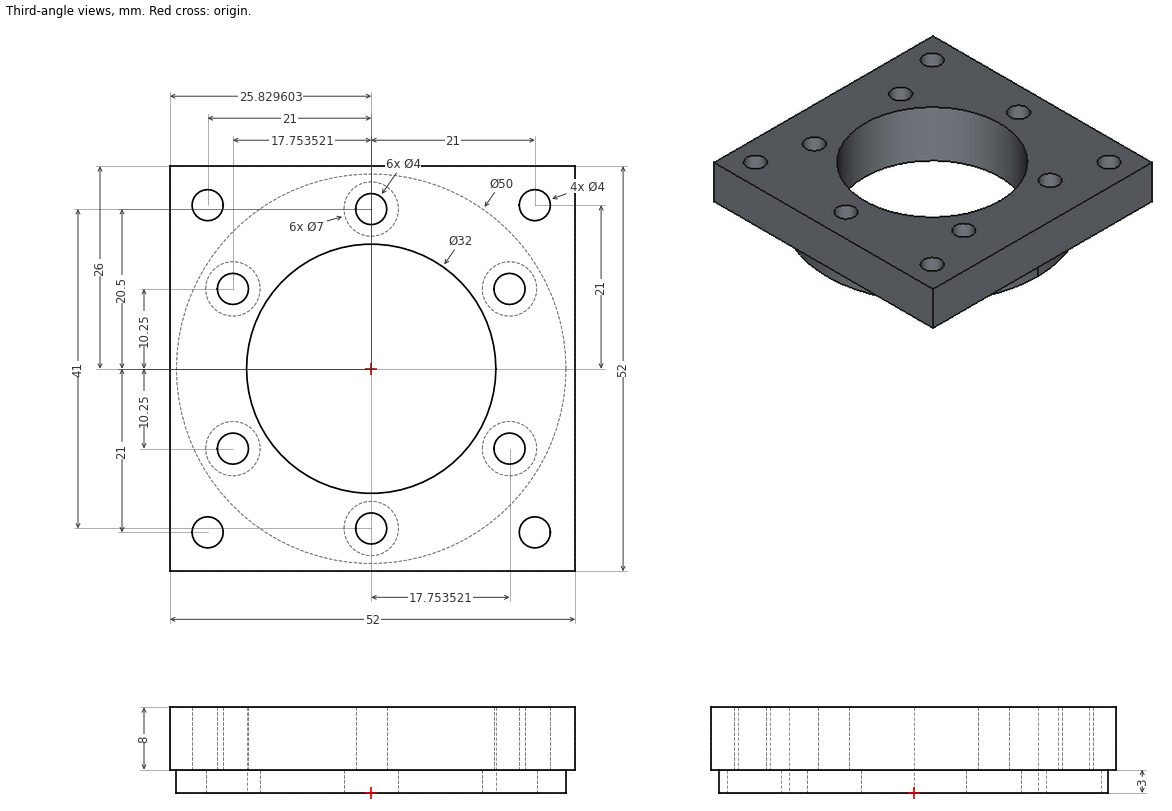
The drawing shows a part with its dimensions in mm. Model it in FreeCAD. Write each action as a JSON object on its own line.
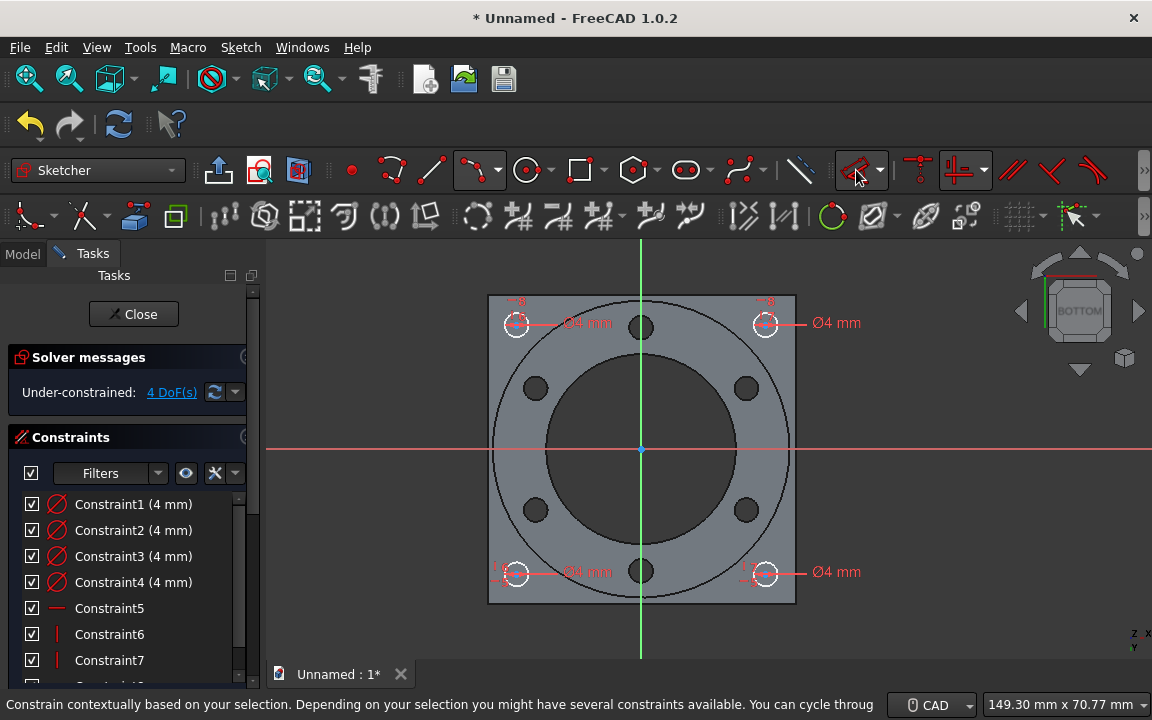
{"action": "left_click", "coordinate": [766, 574]}
{"action": "left_click", "coordinate": [703, 608]}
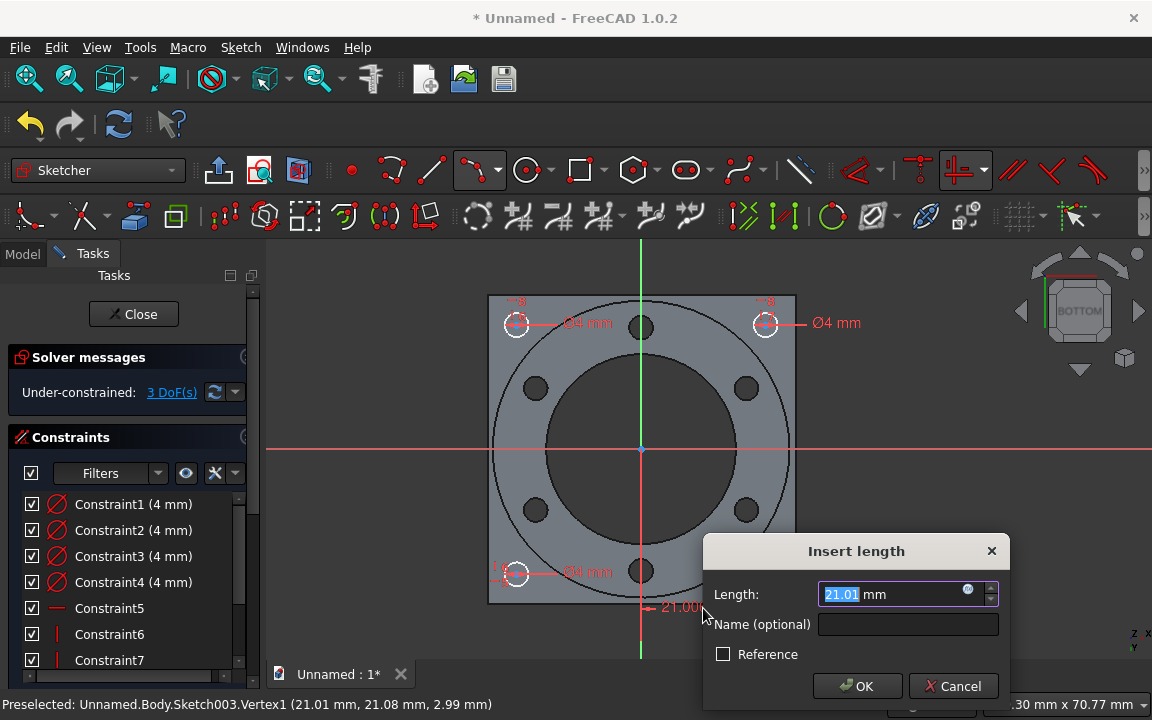
{"action": "type", "text": "21"}
{"action": "key", "text": "Return"}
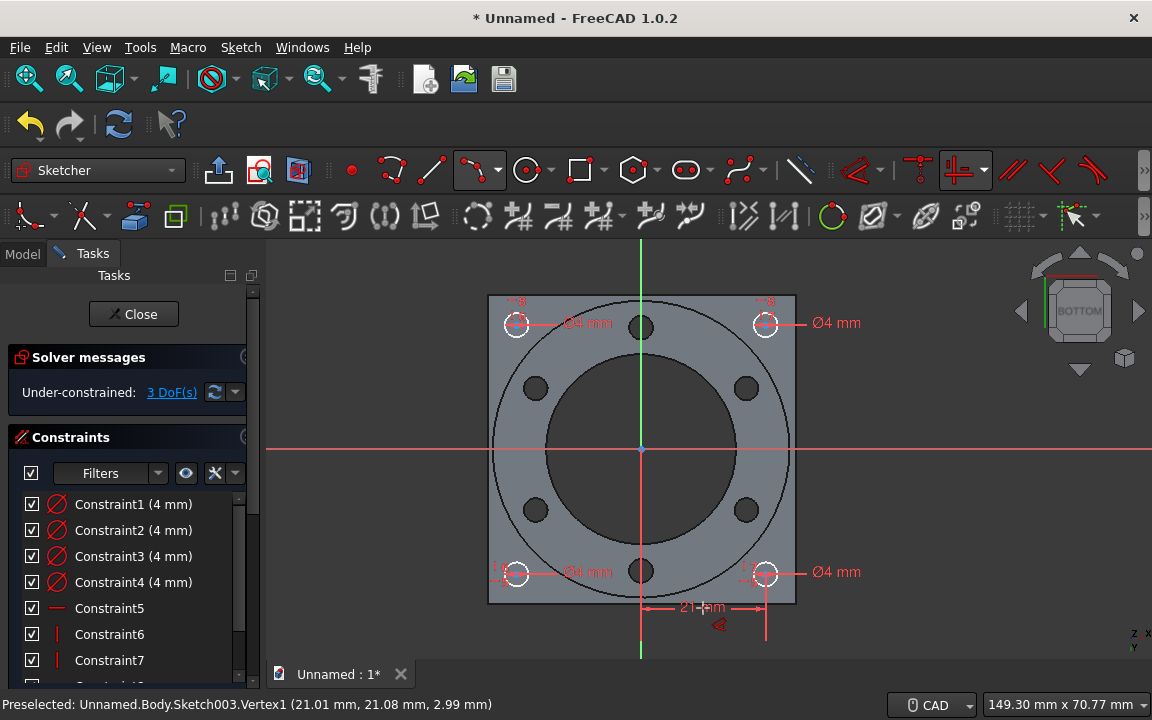
{"action": "left_click", "coordinate": [766, 574]}
{"action": "left_click", "coordinate": [800, 512]}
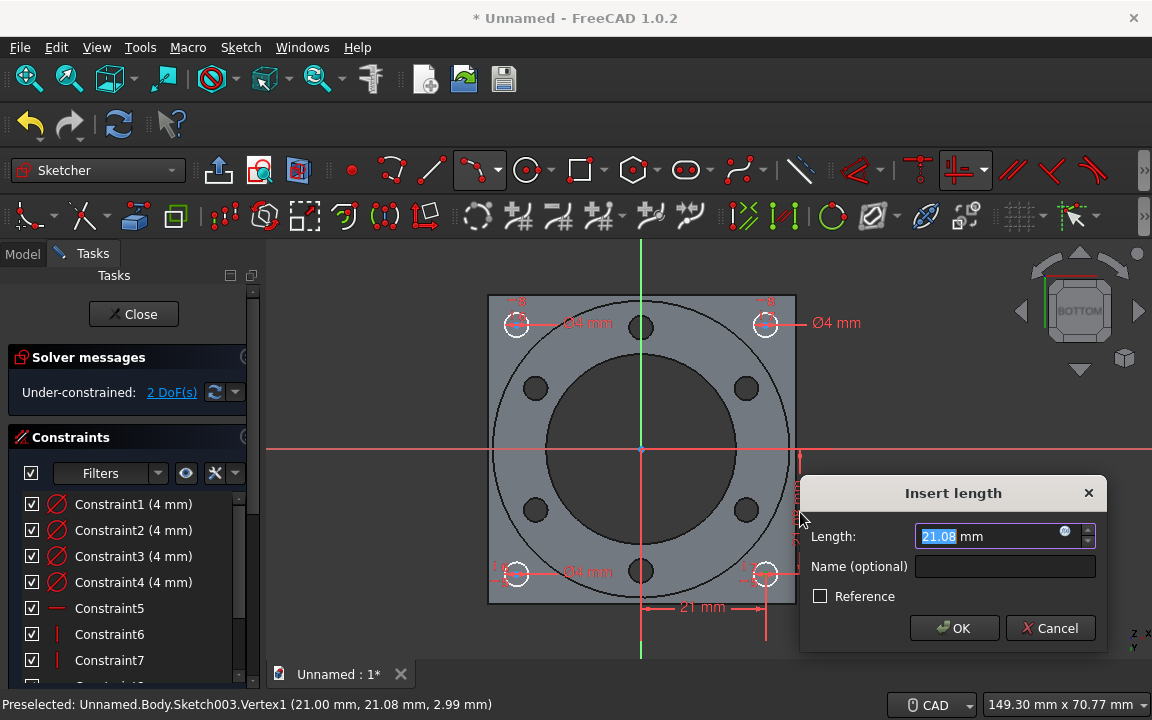
{"action": "type", "text": "21"}
{"action": "key", "text": "Return"}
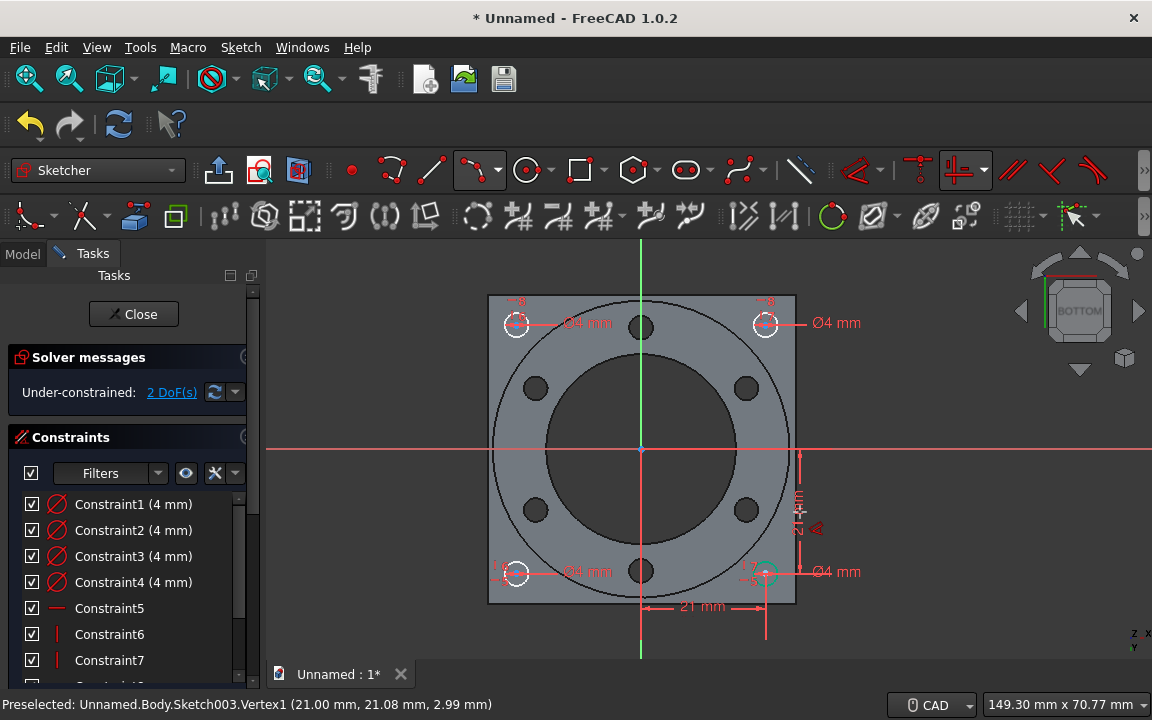
{"action": "left_click", "coordinate": [517, 574]}
{"action": "left_click", "coordinate": [579, 608]}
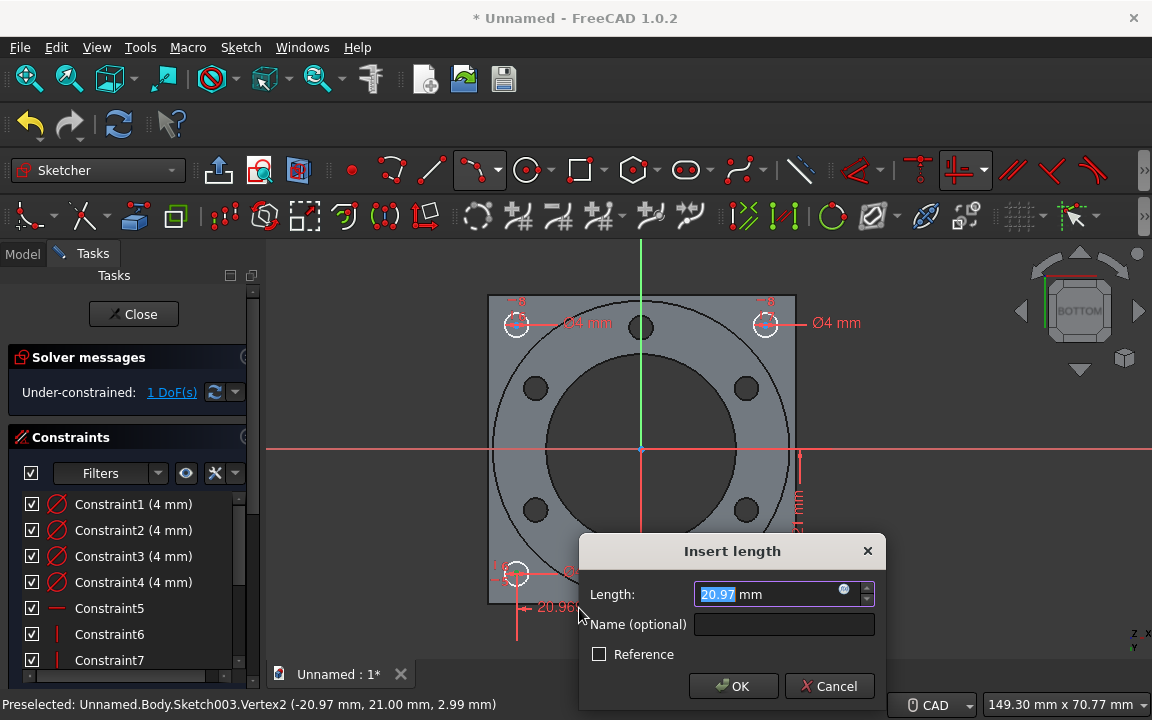
{"action": "type", "text": "21"}
{"action": "key", "text": "Return"}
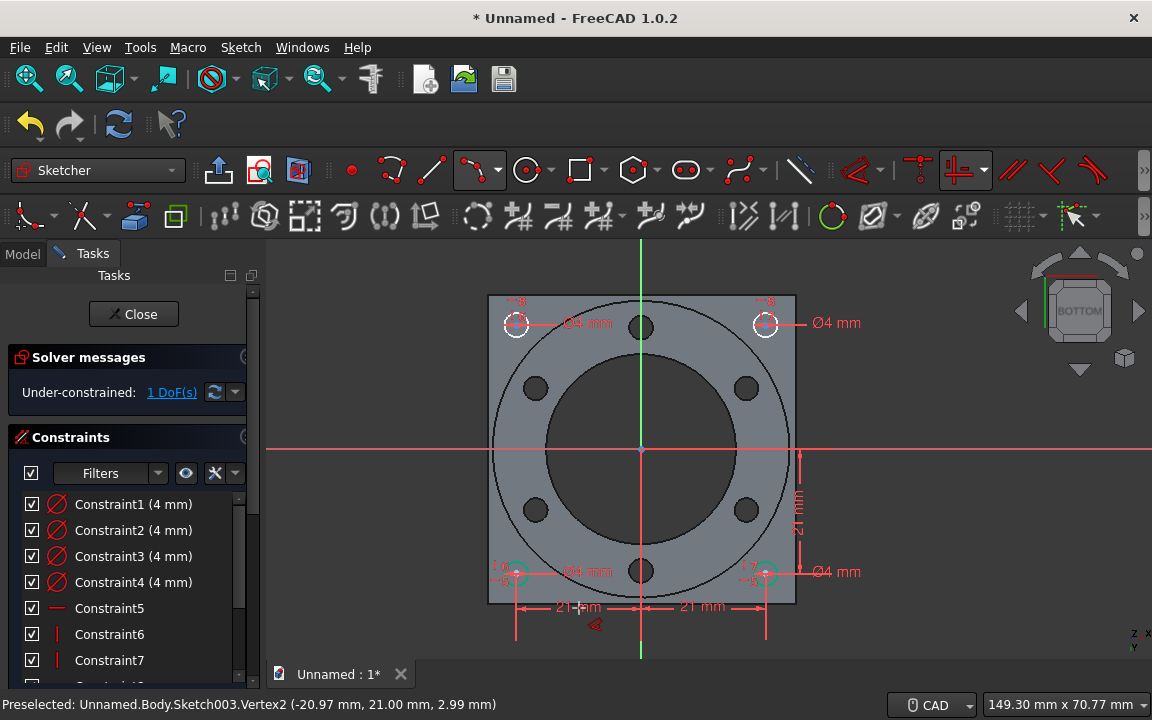
{"action": "left_click", "coordinate": [516, 325]}
{"action": "left_click", "coordinate": [482, 387]}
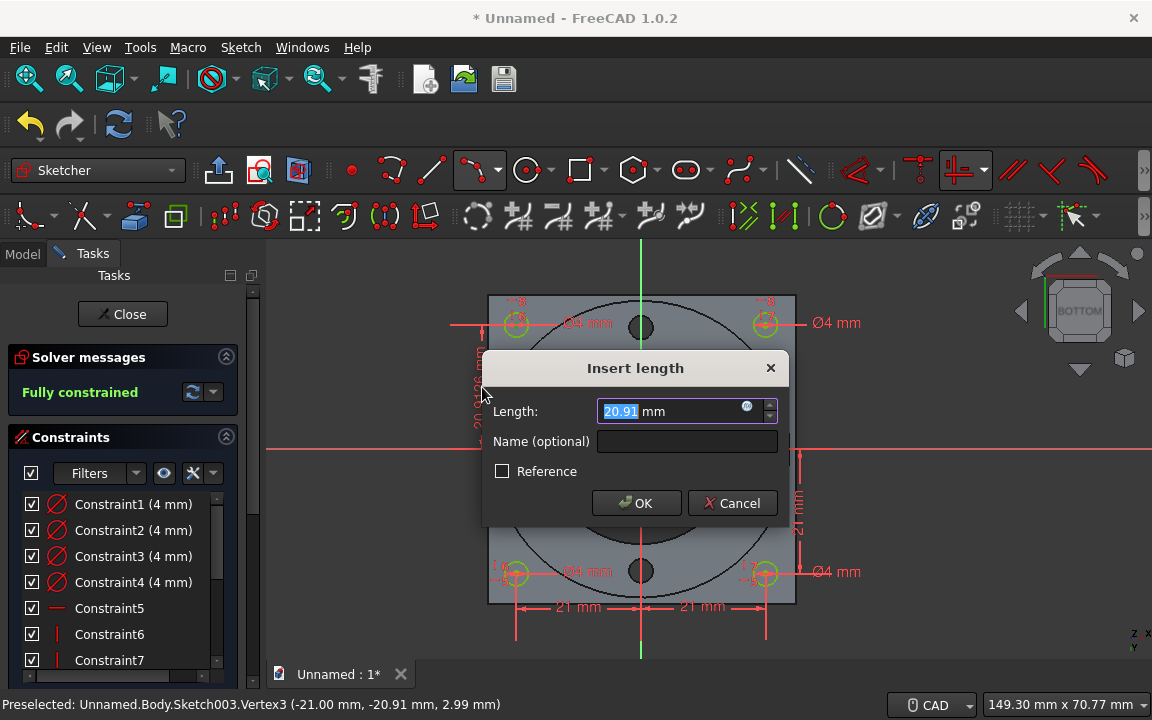
{"action": "type", "text": "21"}
{"action": "key", "text": "Return"}
{"action": "key", "text": "Escape"}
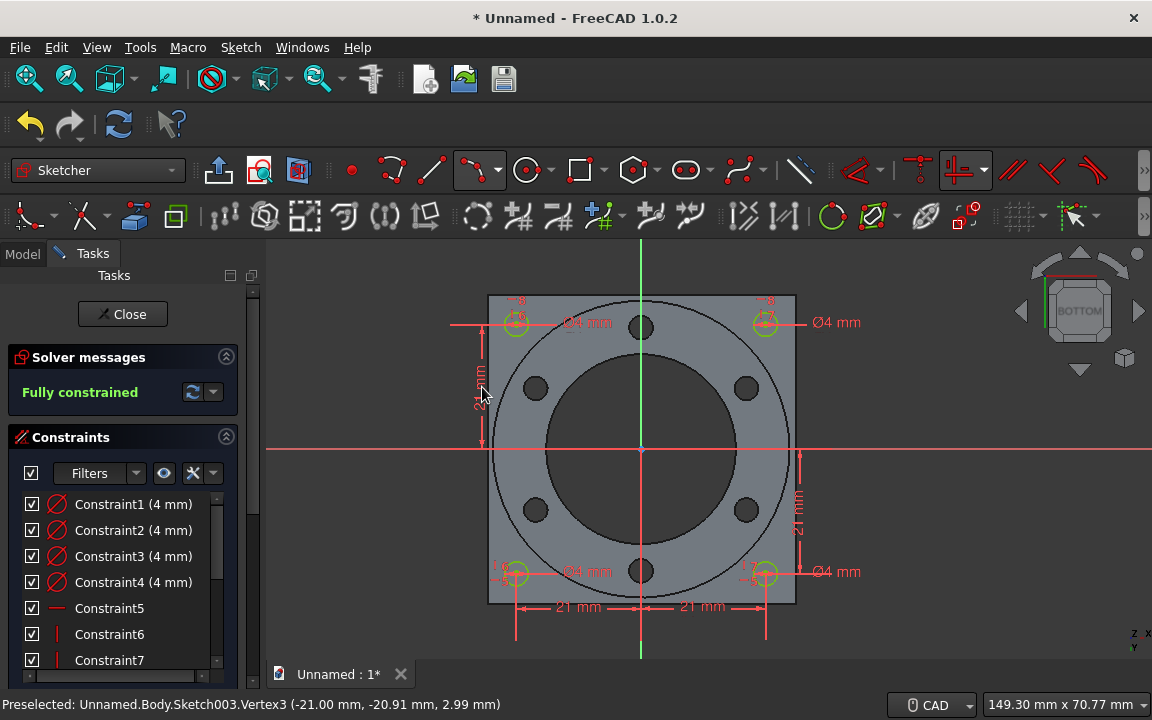
{"action": "left_click", "coordinate": [123, 314]}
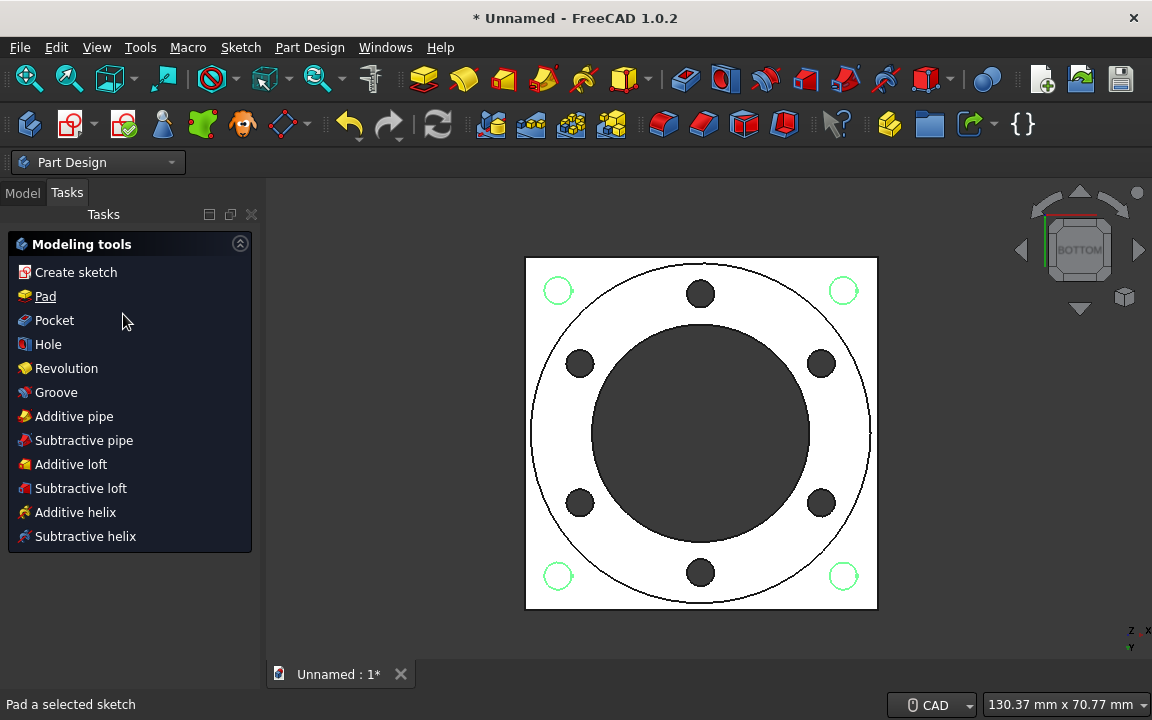
{"action": "left_click", "coordinate": [686, 80]}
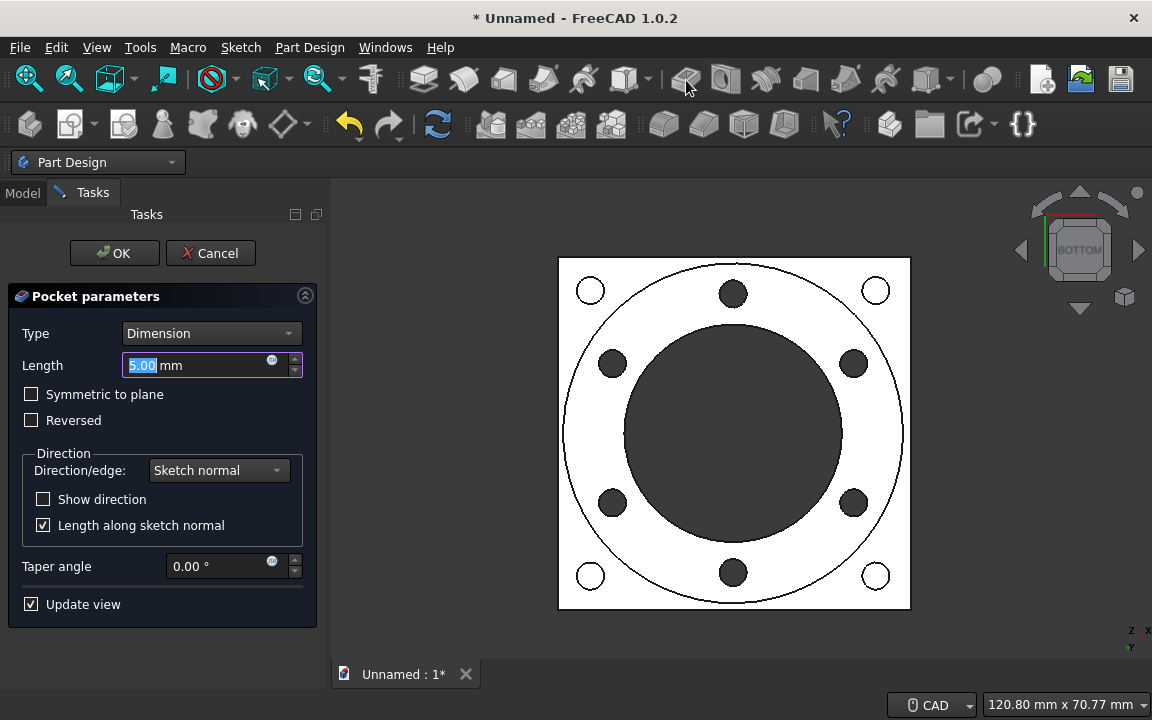
{"action": "left_click", "coordinate": [212, 334]}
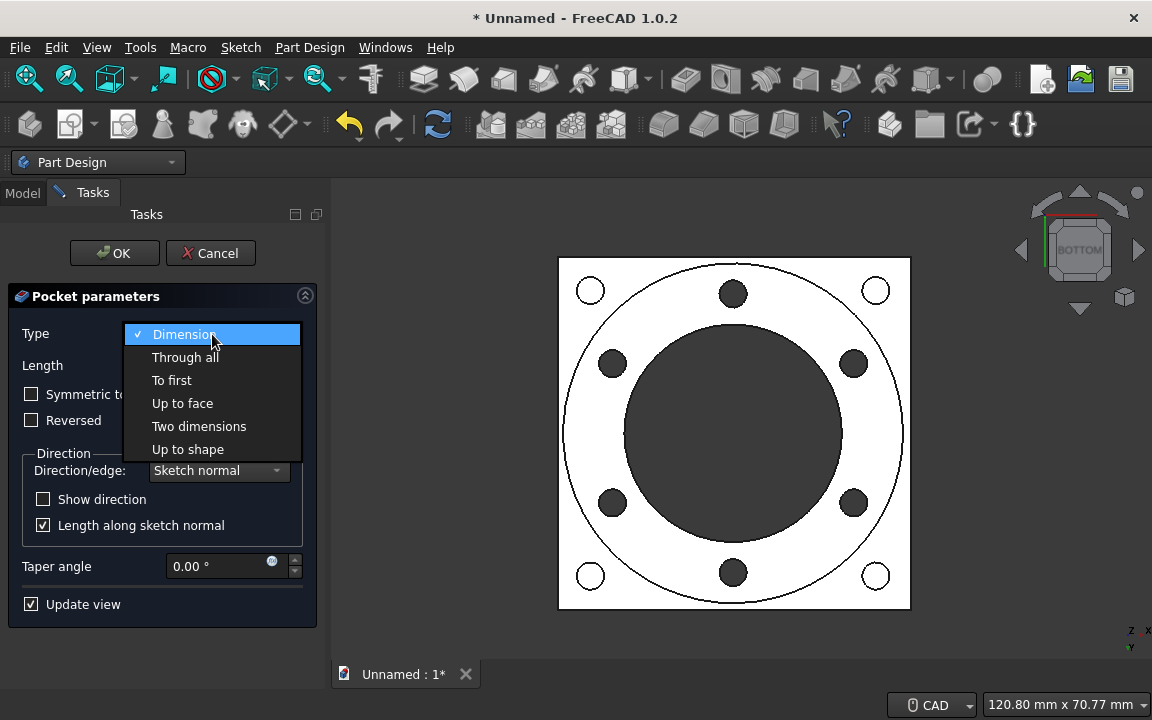
{"action": "left_click", "coordinate": [212, 358]}